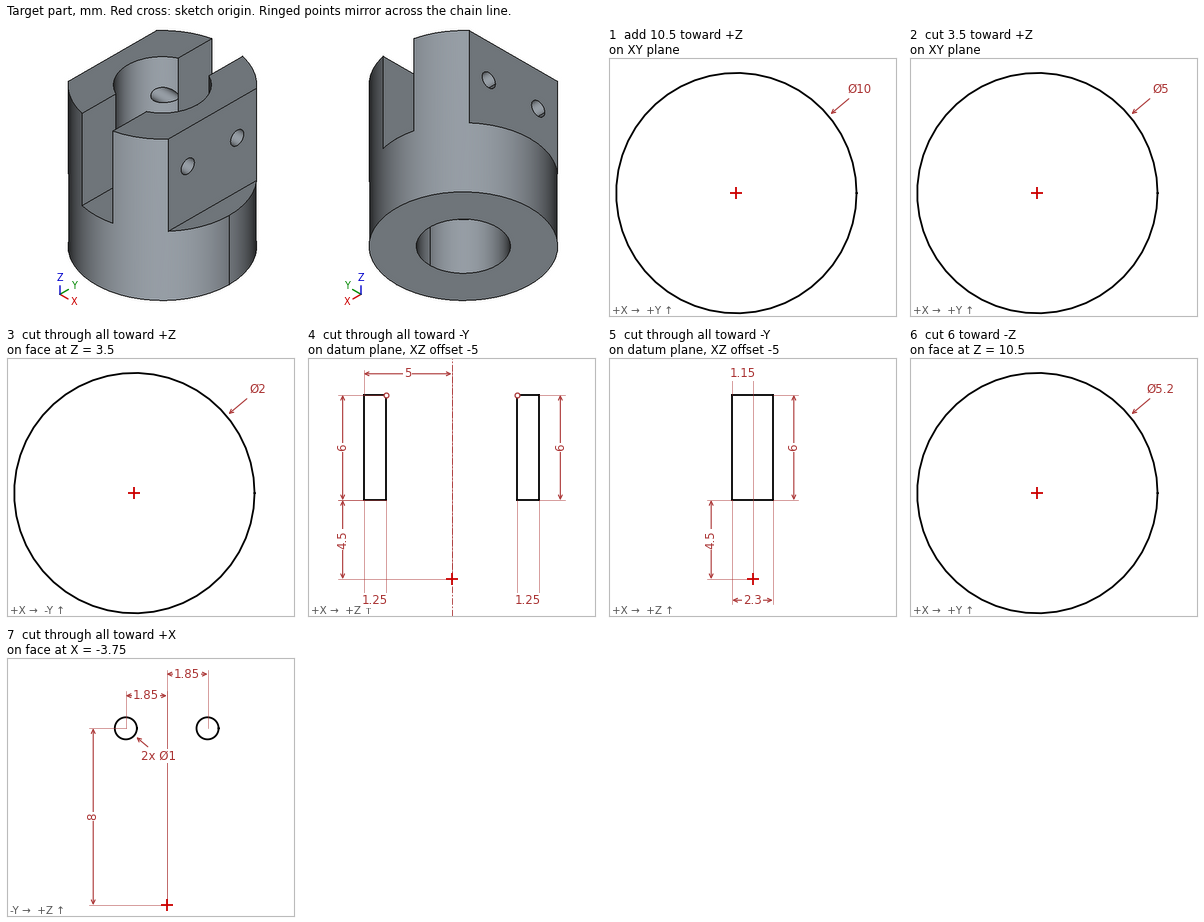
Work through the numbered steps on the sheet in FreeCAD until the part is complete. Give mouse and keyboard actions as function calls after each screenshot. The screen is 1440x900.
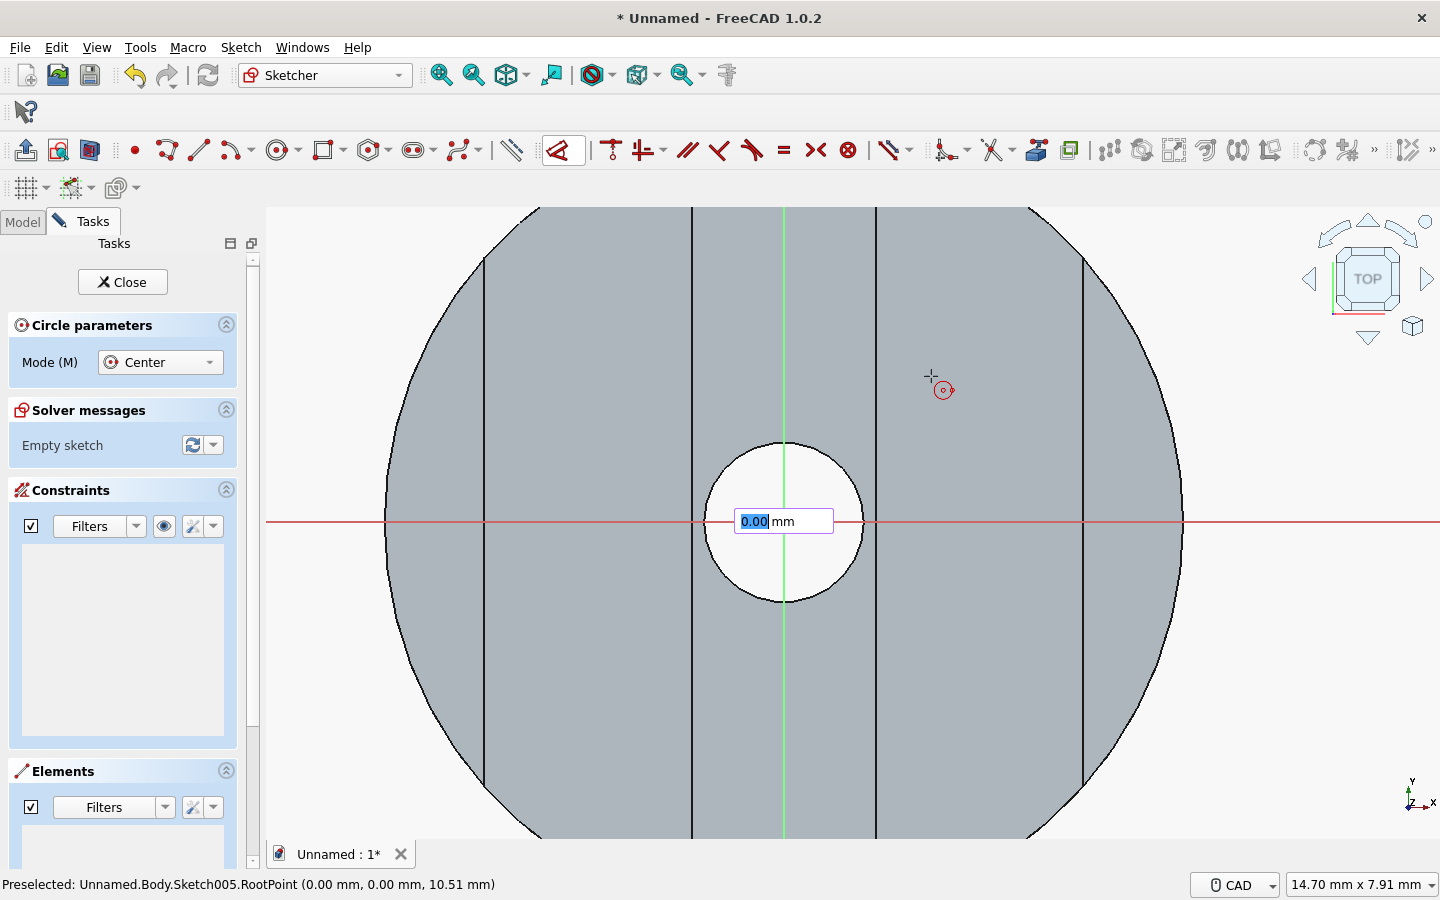
text(5.2)
key(Return)
key(Escape)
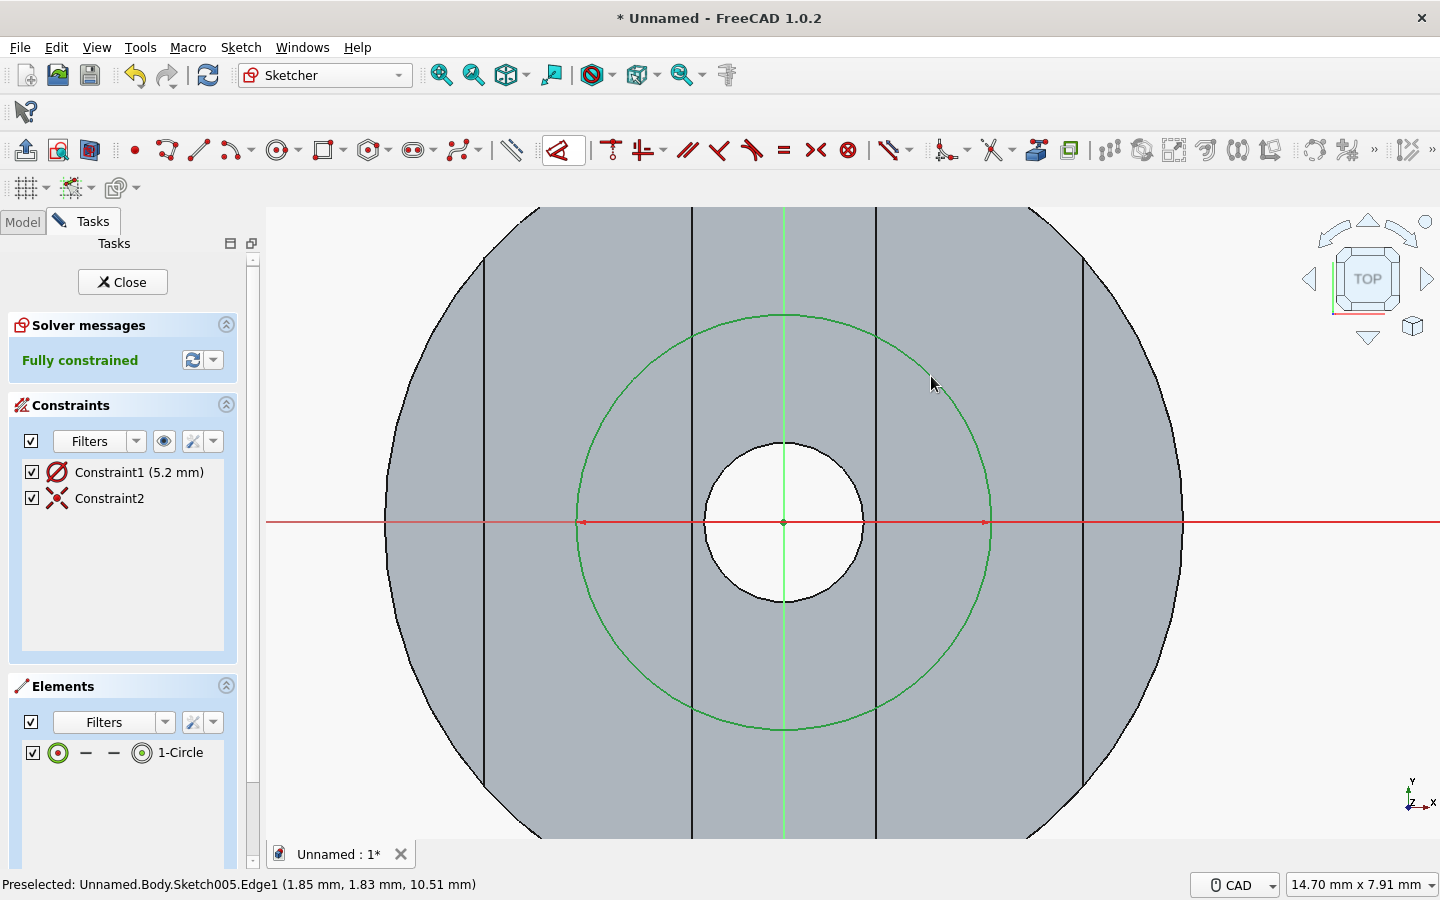
click(123, 282)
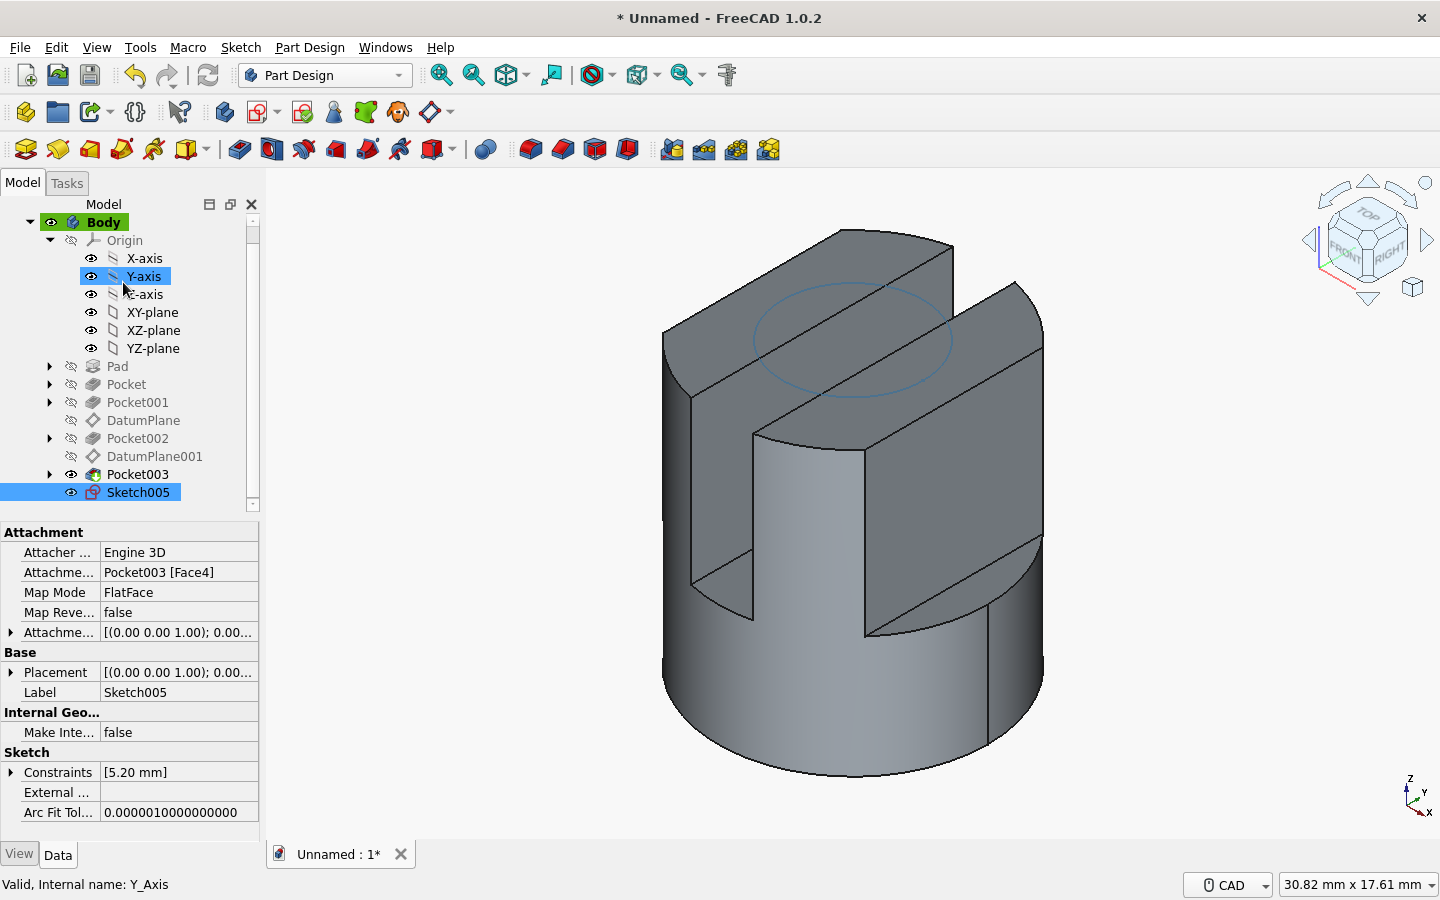
click(240, 150)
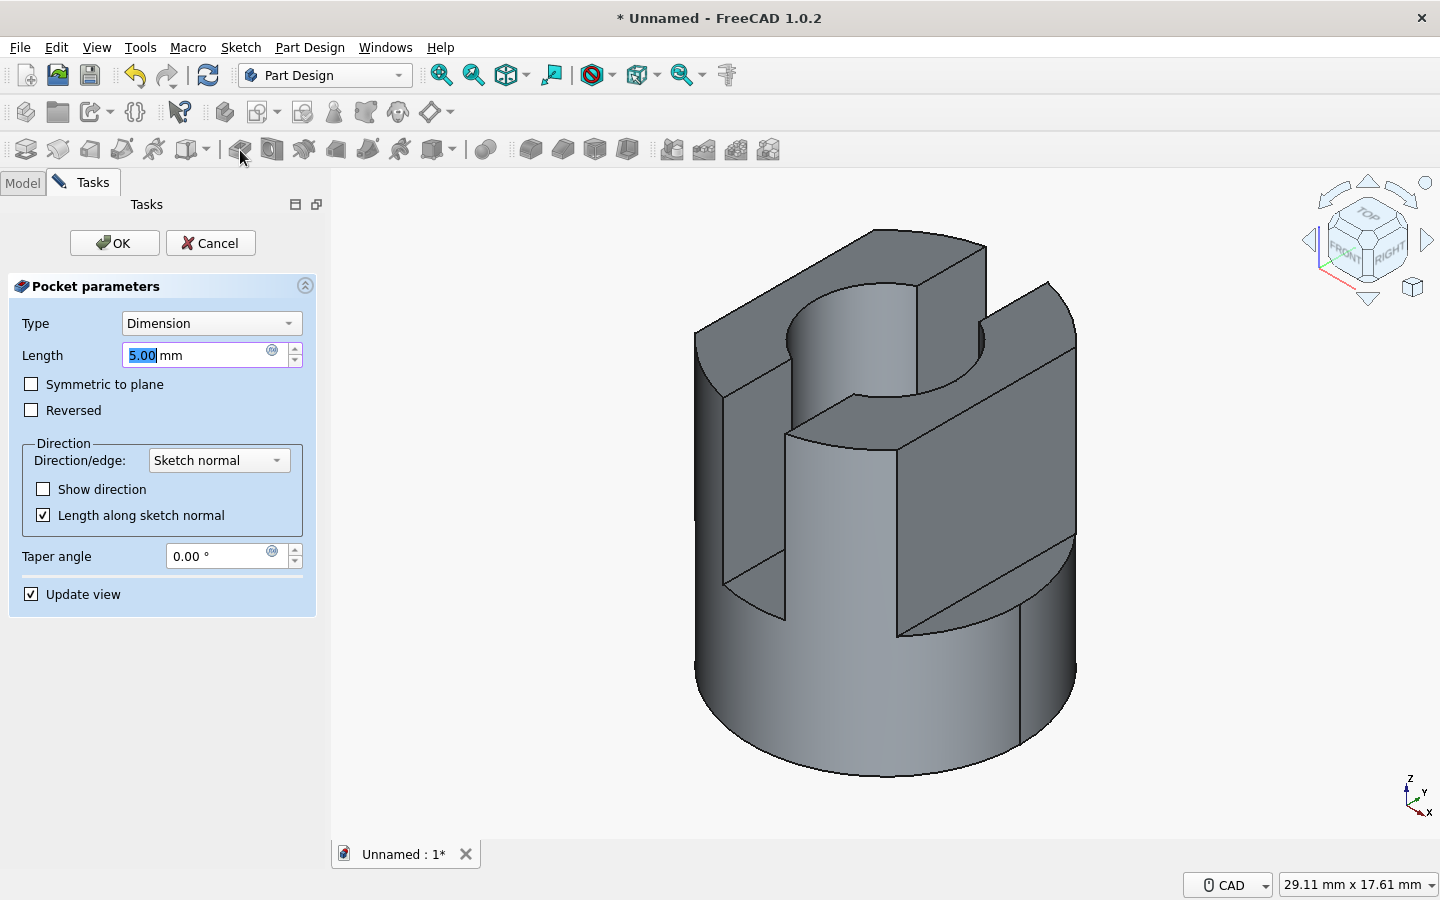
text(6)
key(Tab)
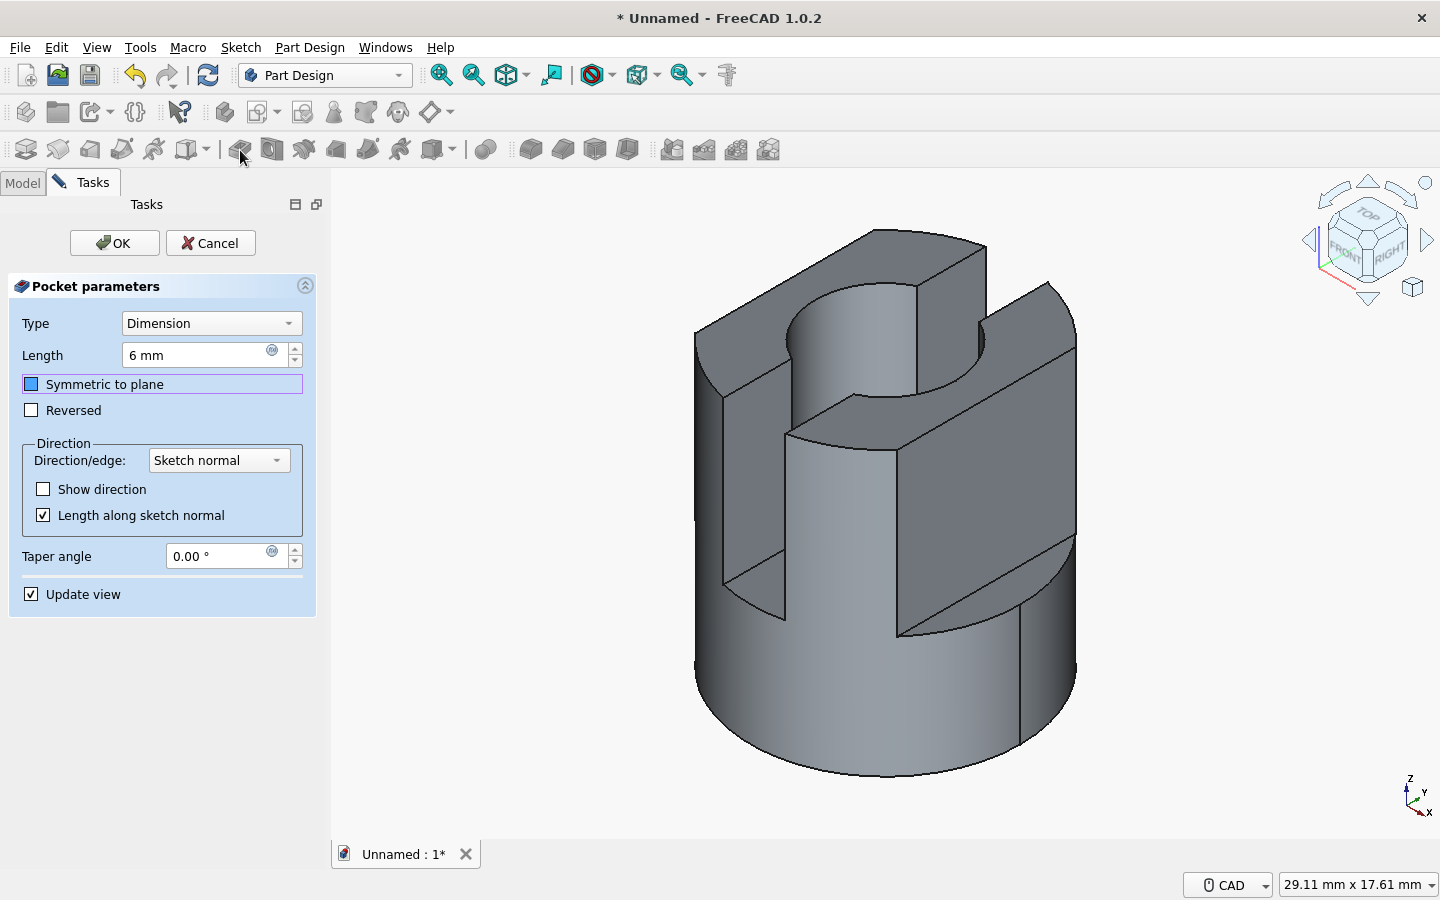
click(115, 243)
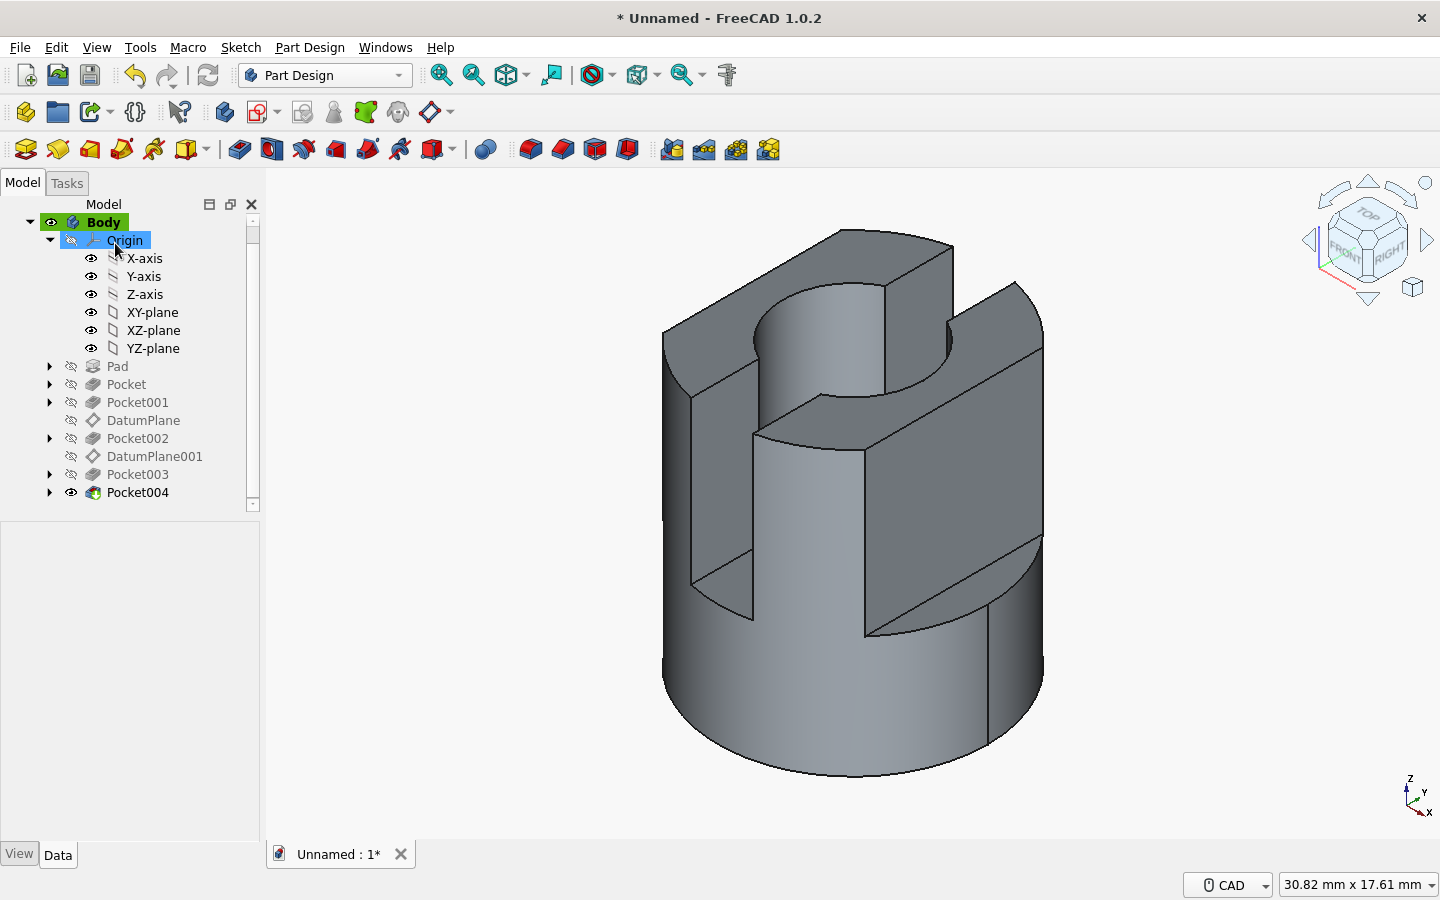
key(6)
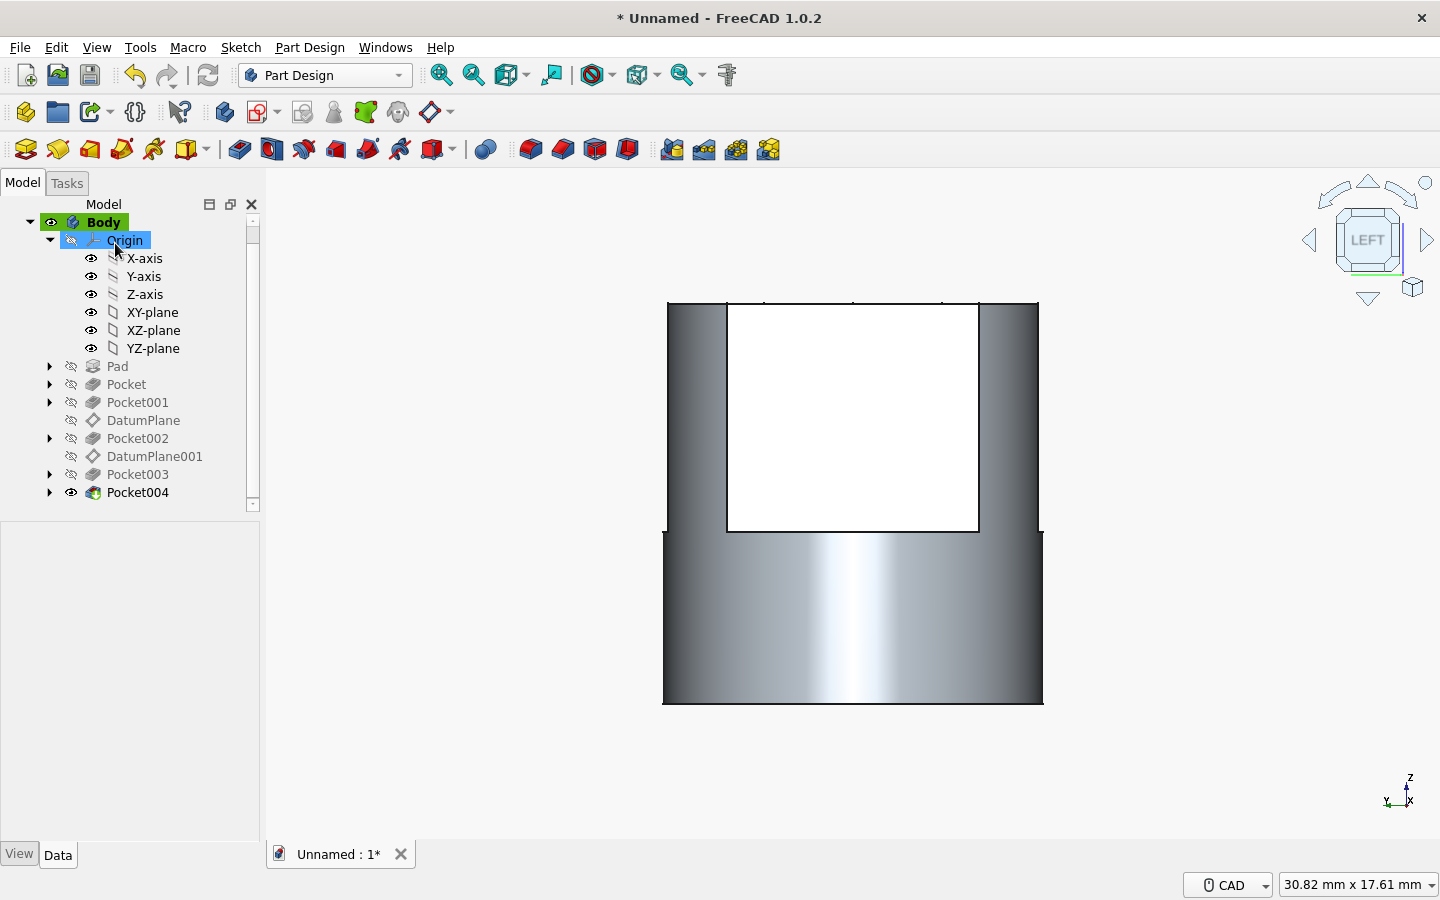
click(853, 417)